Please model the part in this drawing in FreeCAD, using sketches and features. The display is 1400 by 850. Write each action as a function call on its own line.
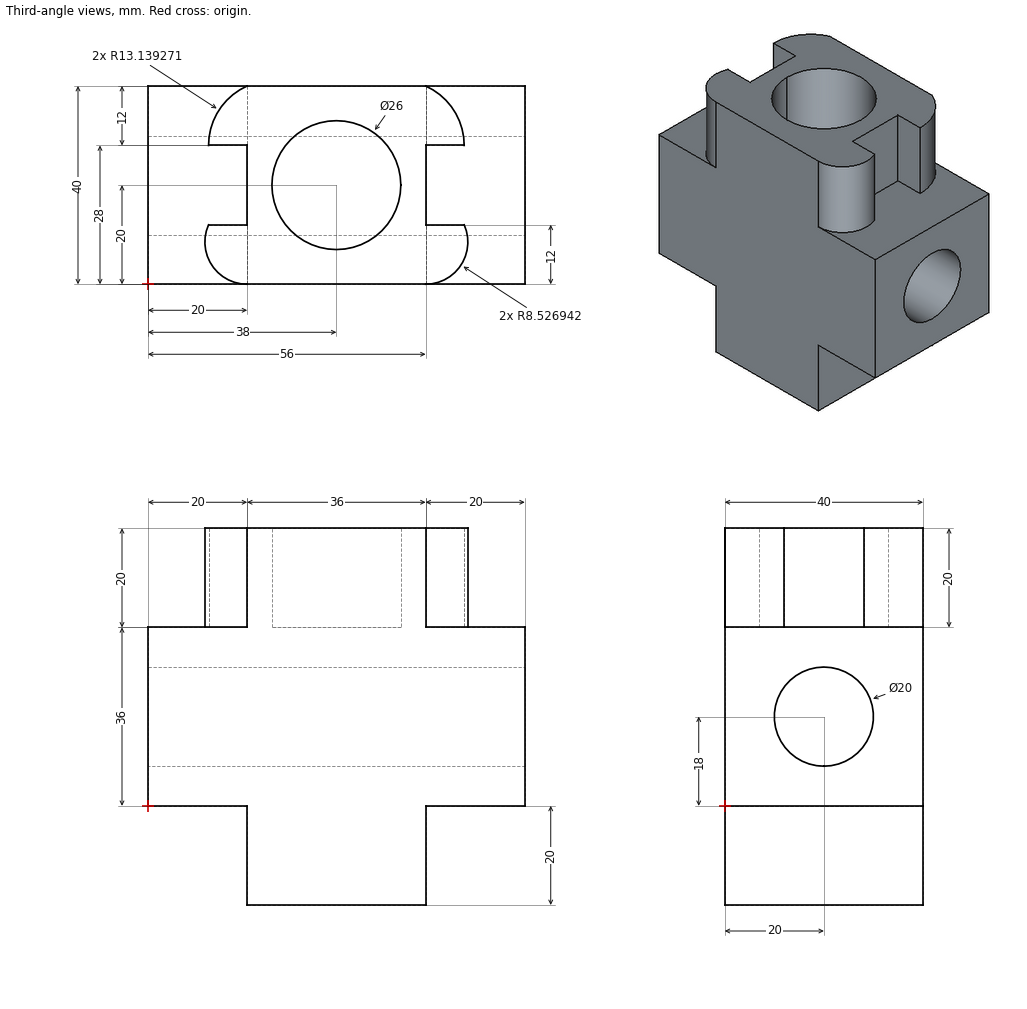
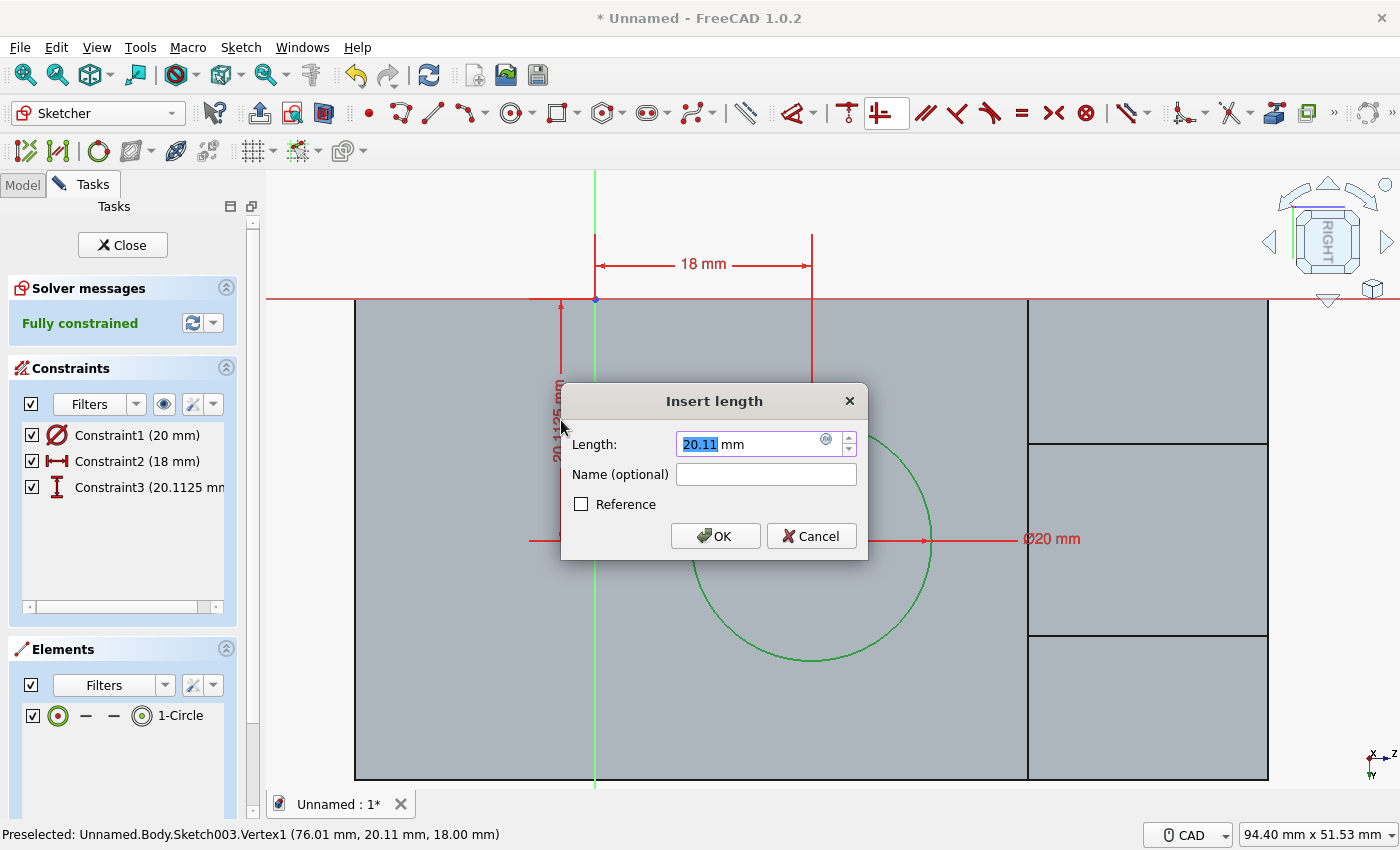
text(20)
key(Return)
key(Escape)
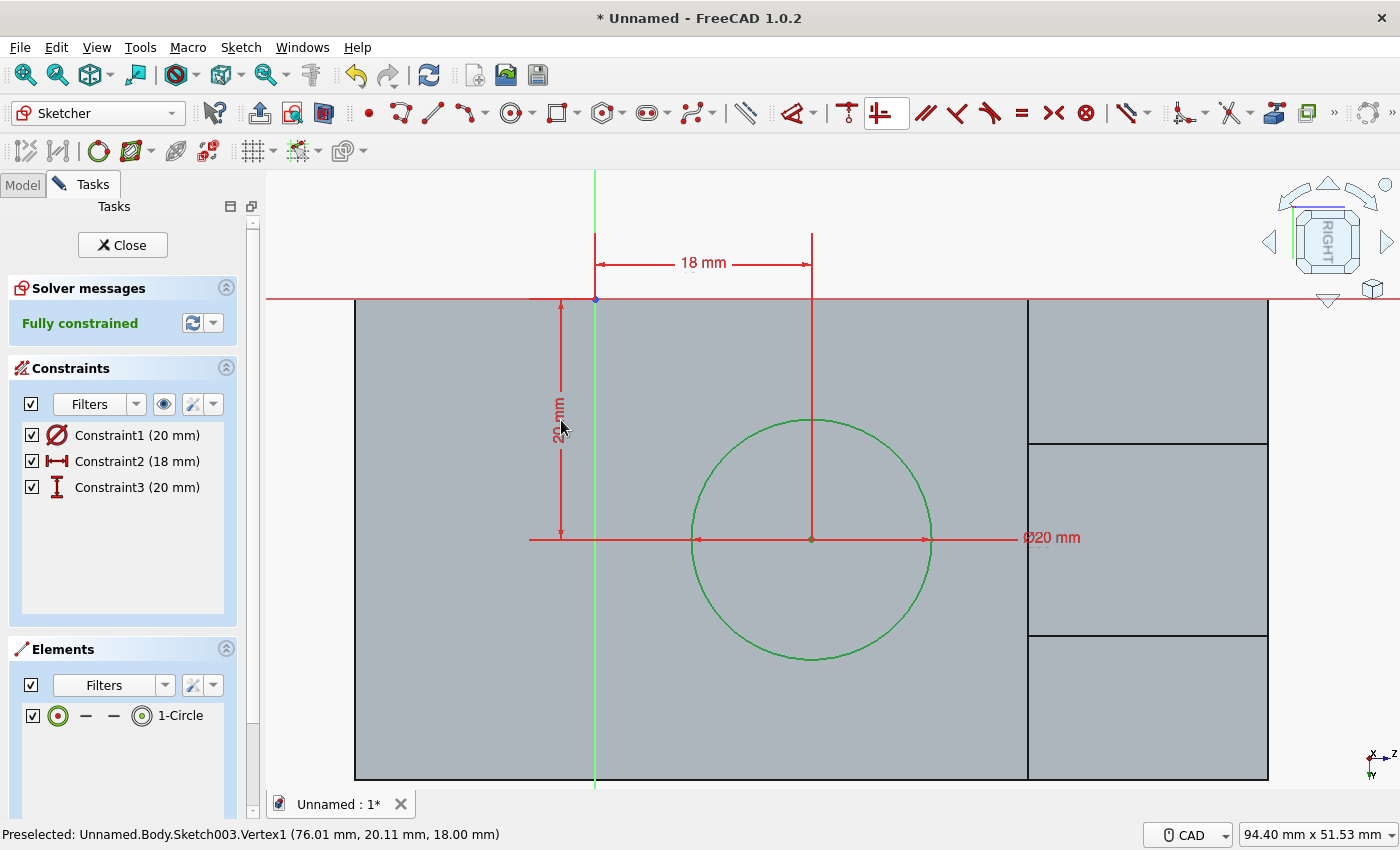
click(123, 245)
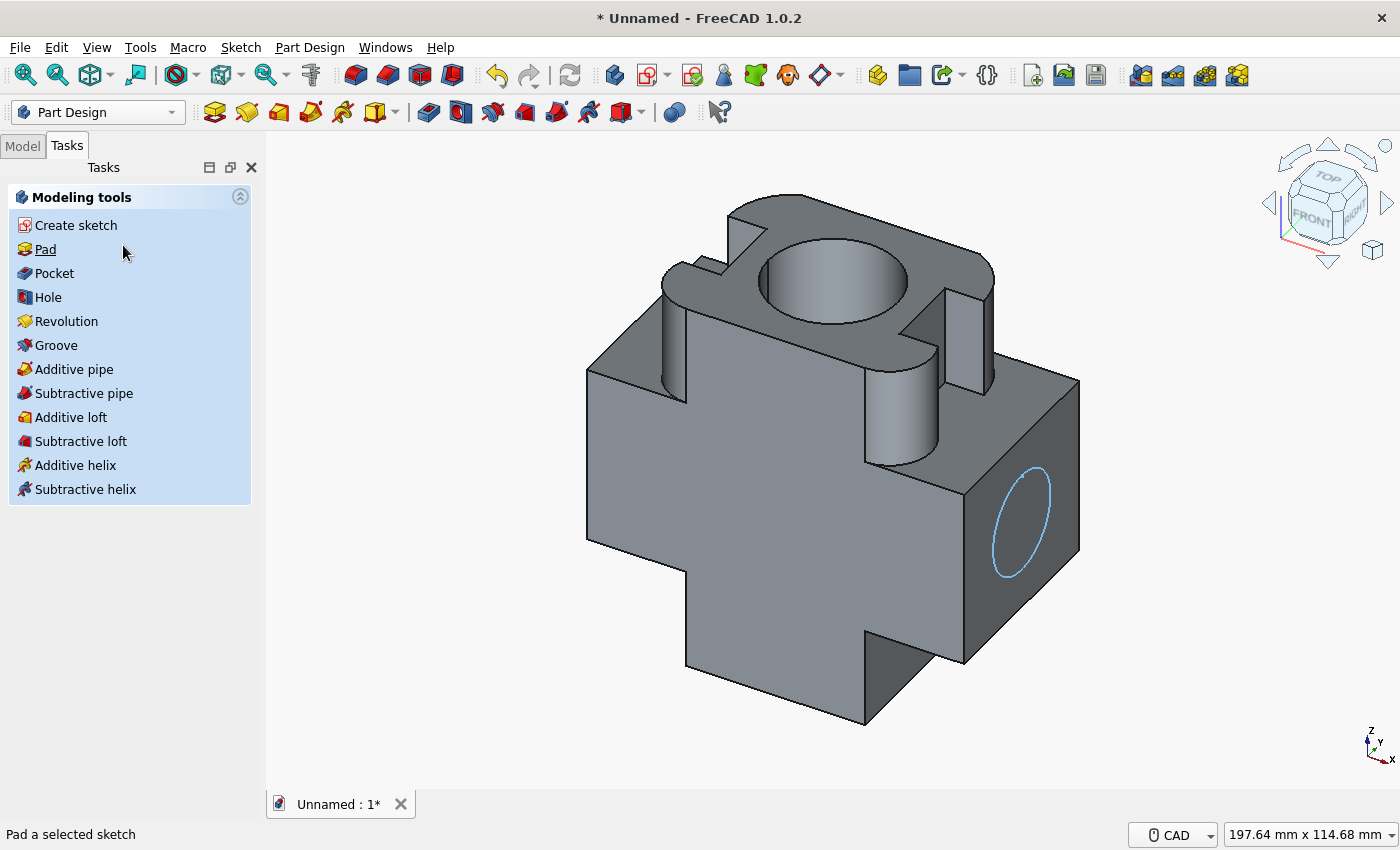
click(430, 112)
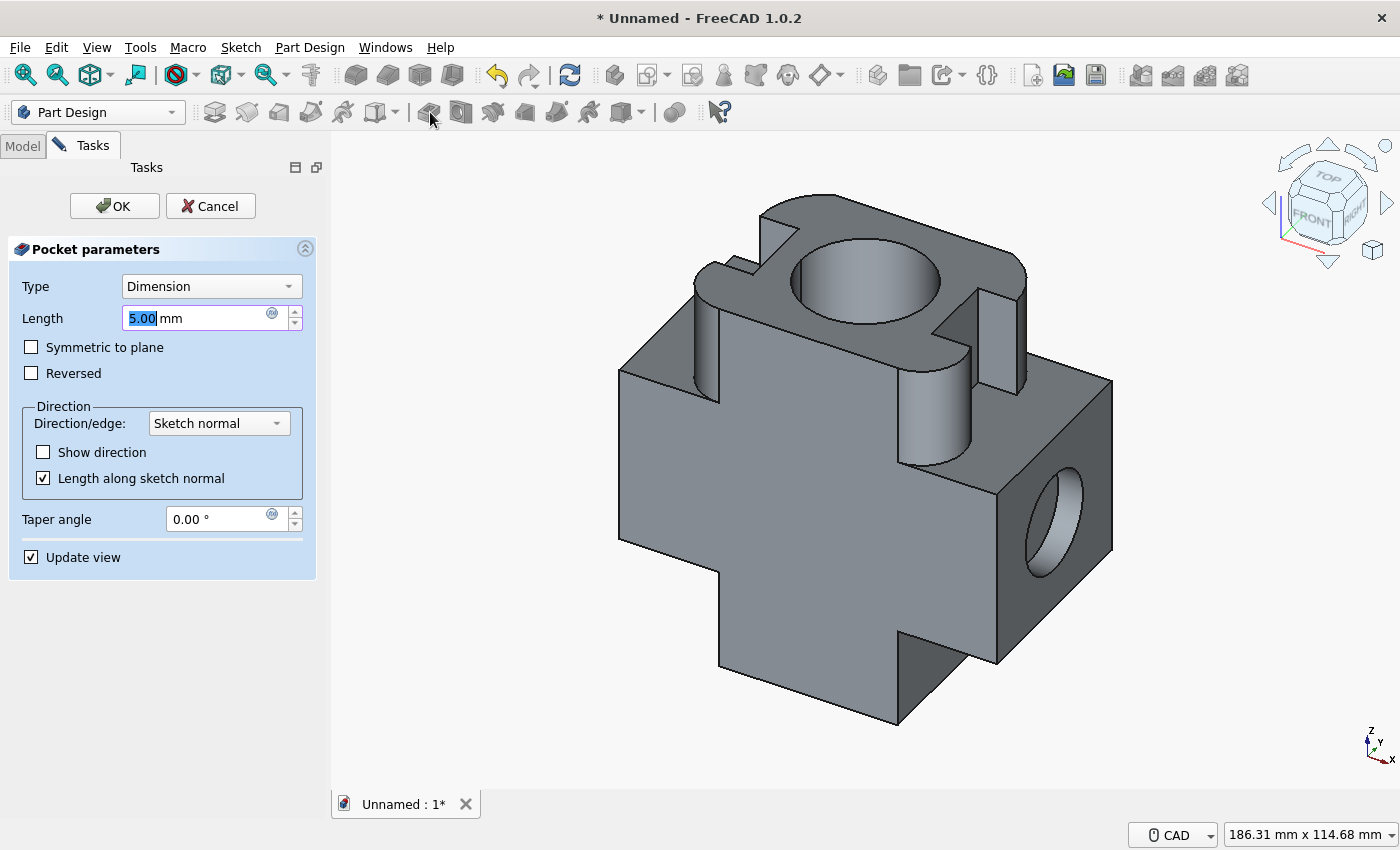
click(212, 286)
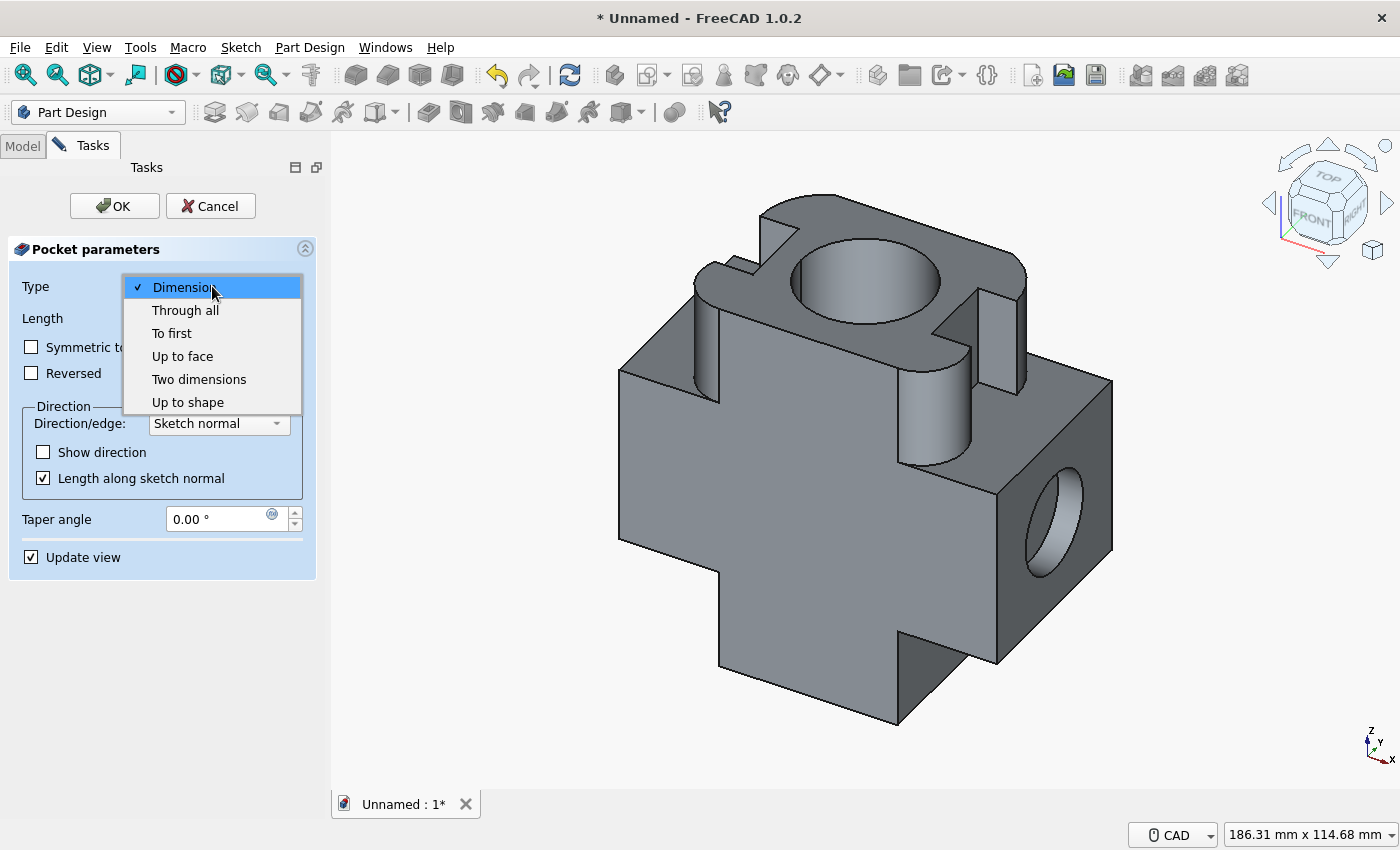
click(212, 310)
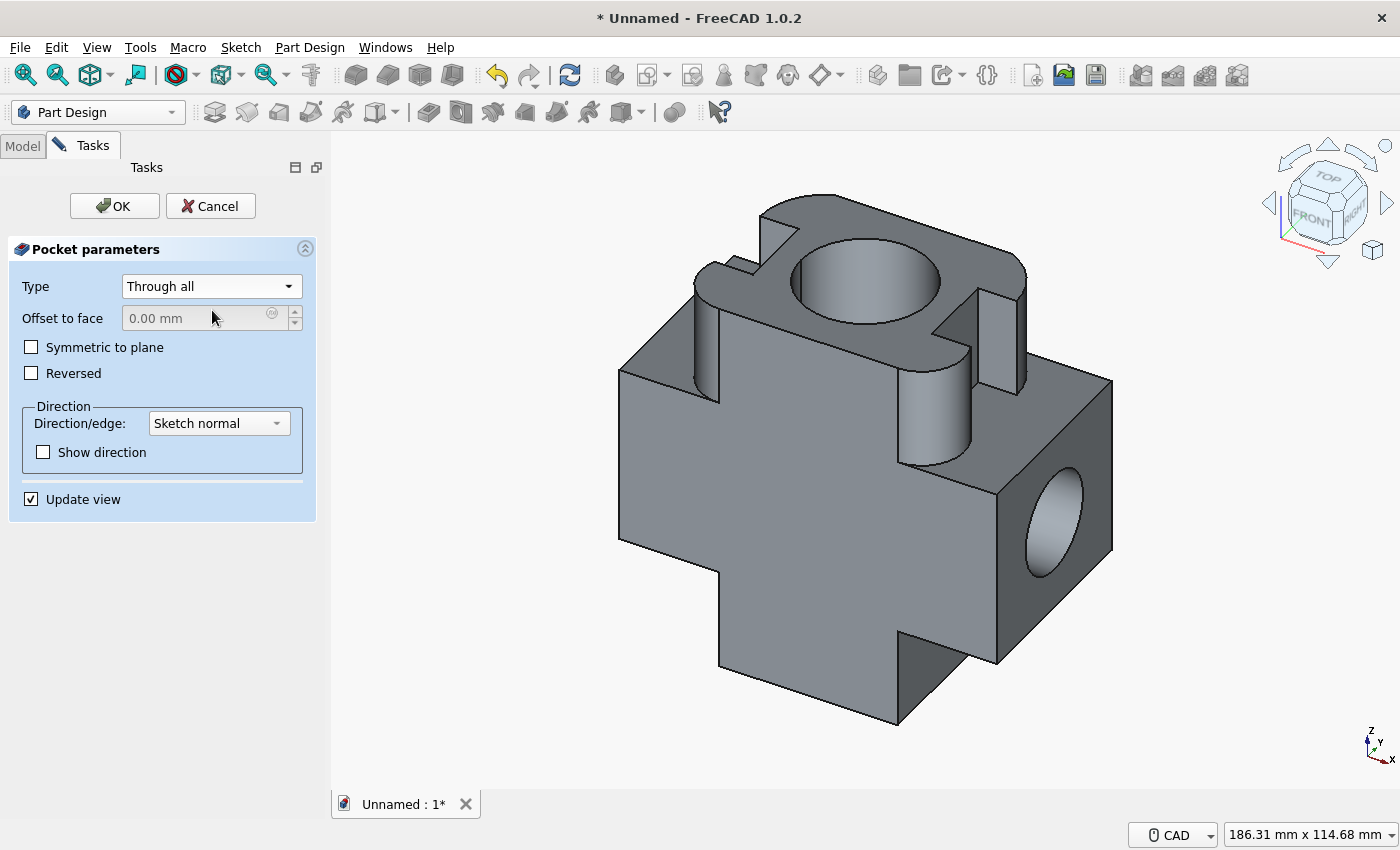
click(115, 206)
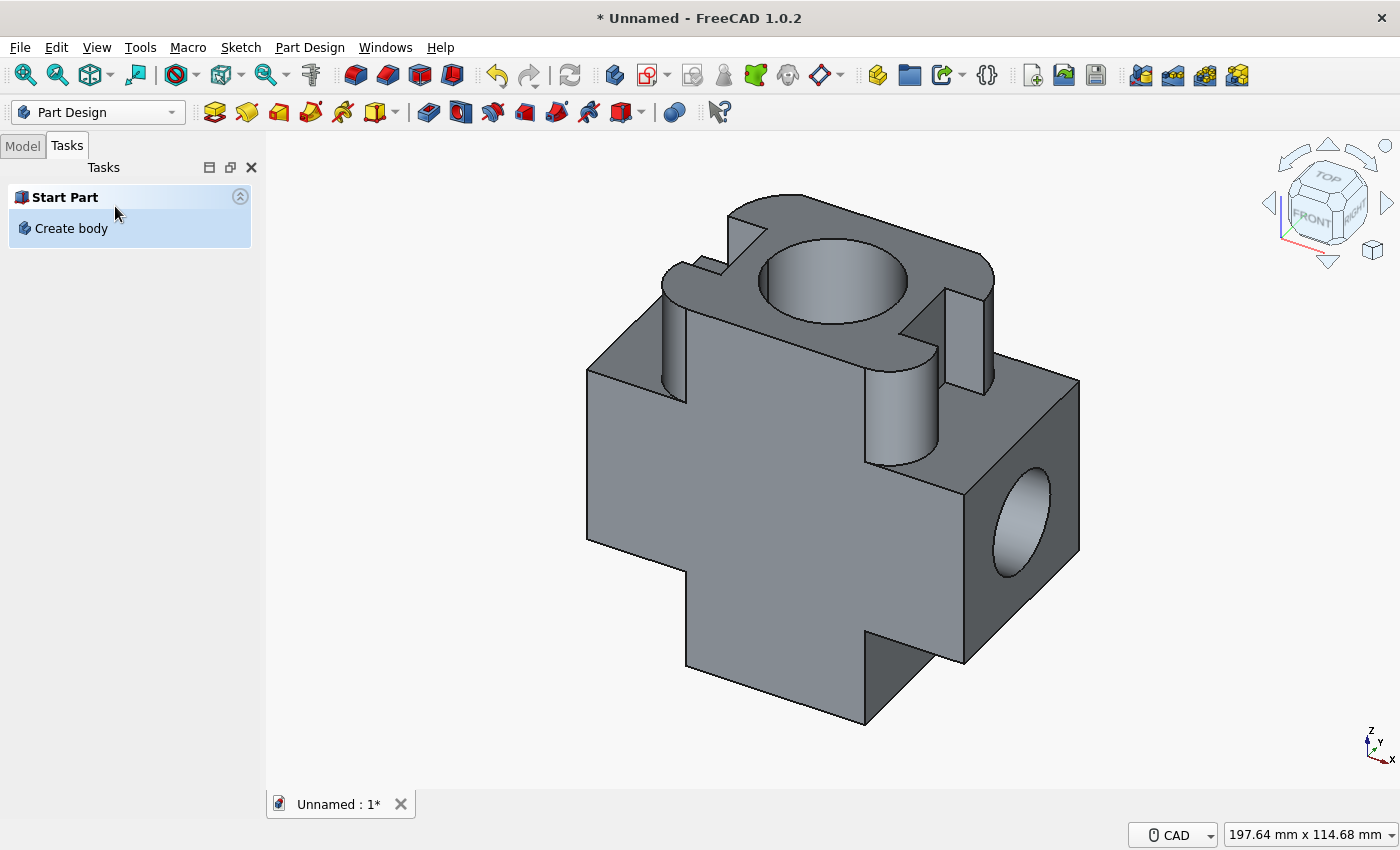
key(0)